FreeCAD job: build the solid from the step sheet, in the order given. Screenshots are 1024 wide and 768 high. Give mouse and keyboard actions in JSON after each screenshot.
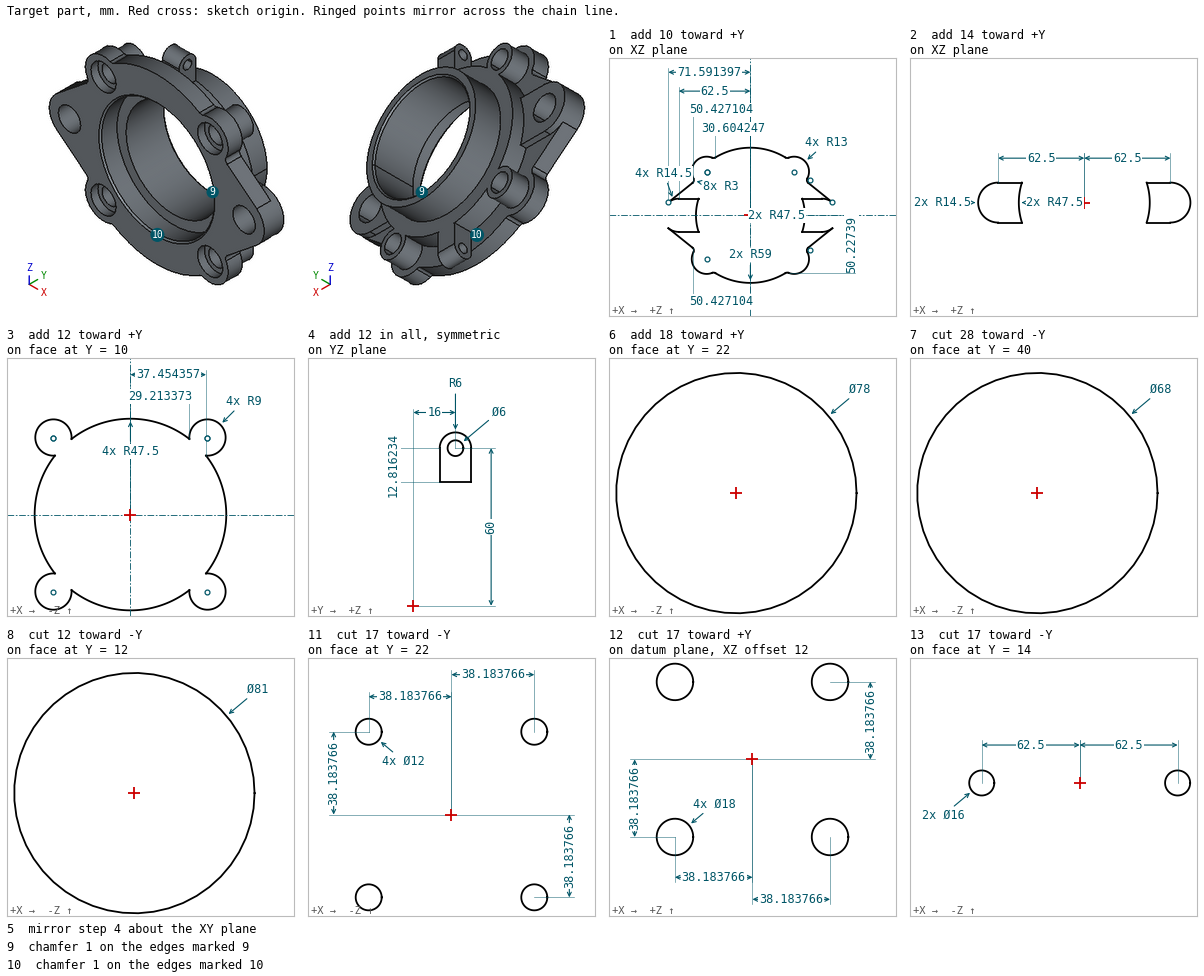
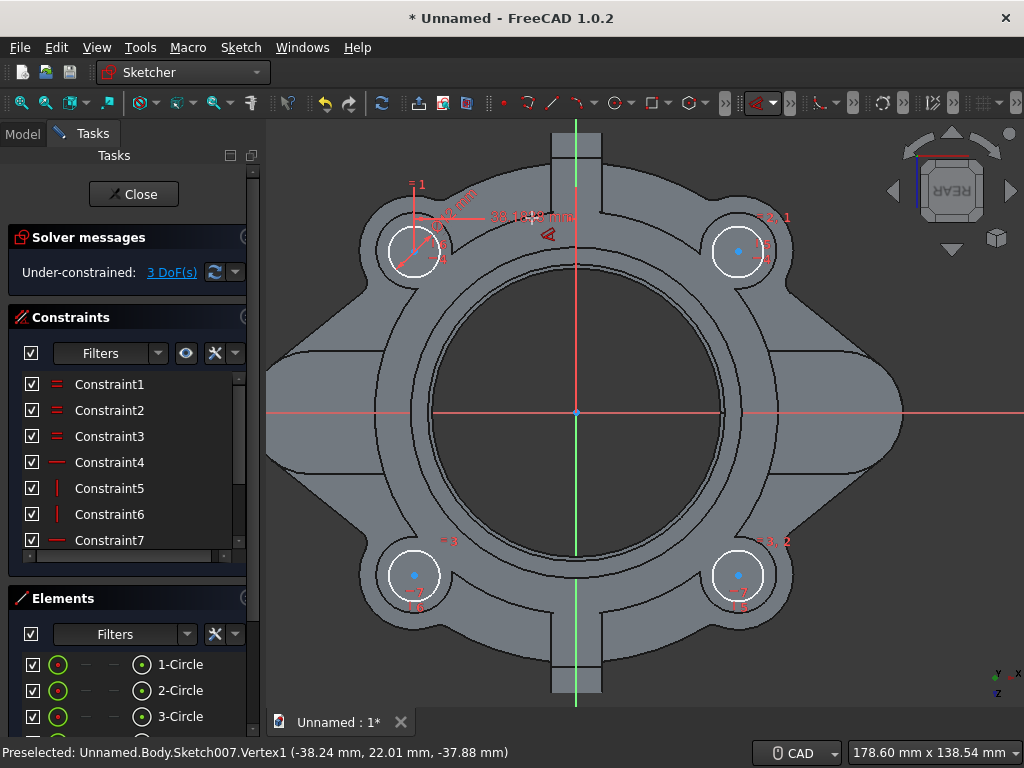
{"action": "left_click", "coordinate": [414, 252]}
{"action": "left_click", "coordinate": [380, 332]}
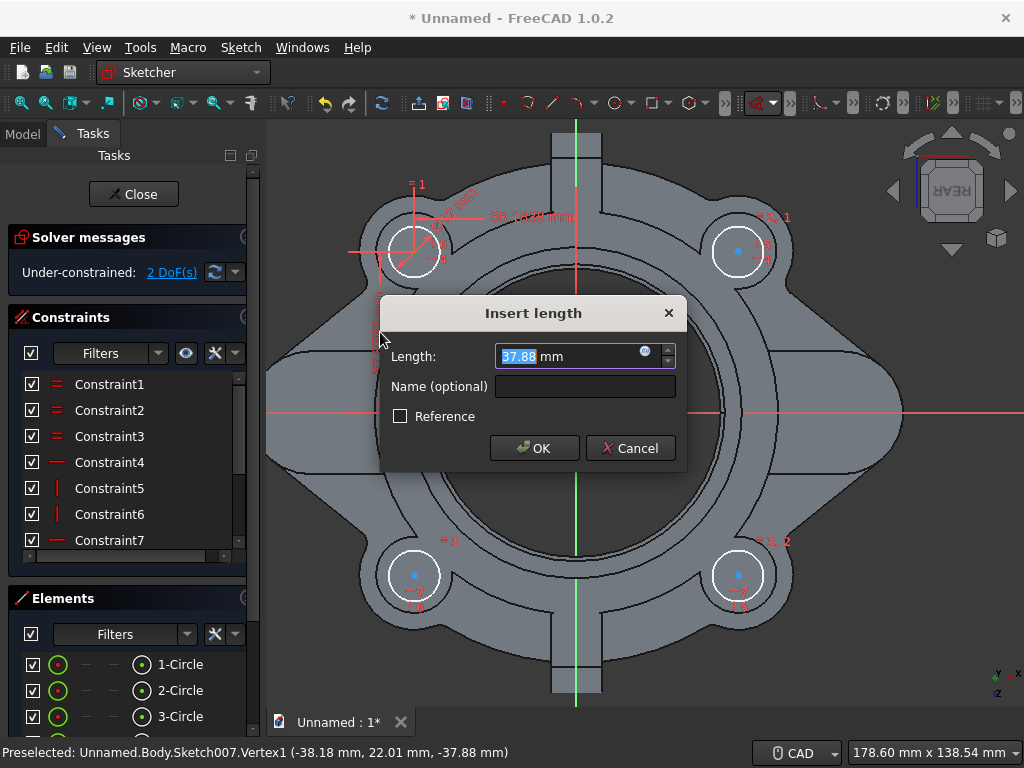
{"action": "type", "text": "38.183766"}
{"action": "key", "text": "Return"}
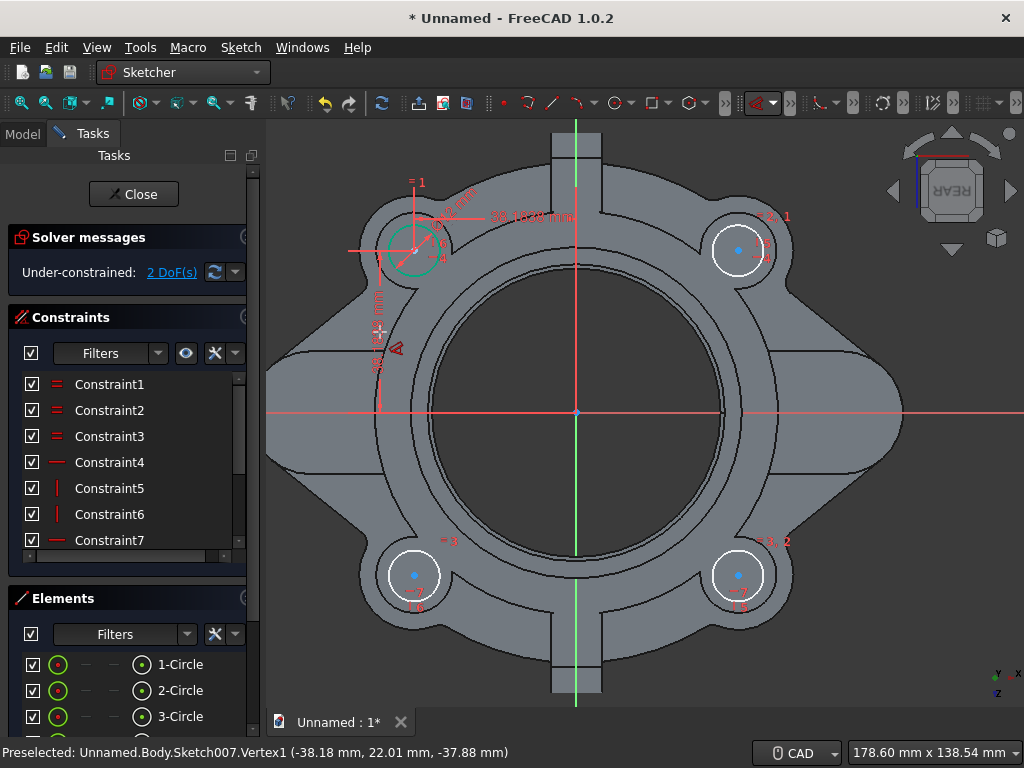
{"action": "left_click", "coordinate": [738, 251]}
{"action": "left_click", "coordinate": [657, 217]}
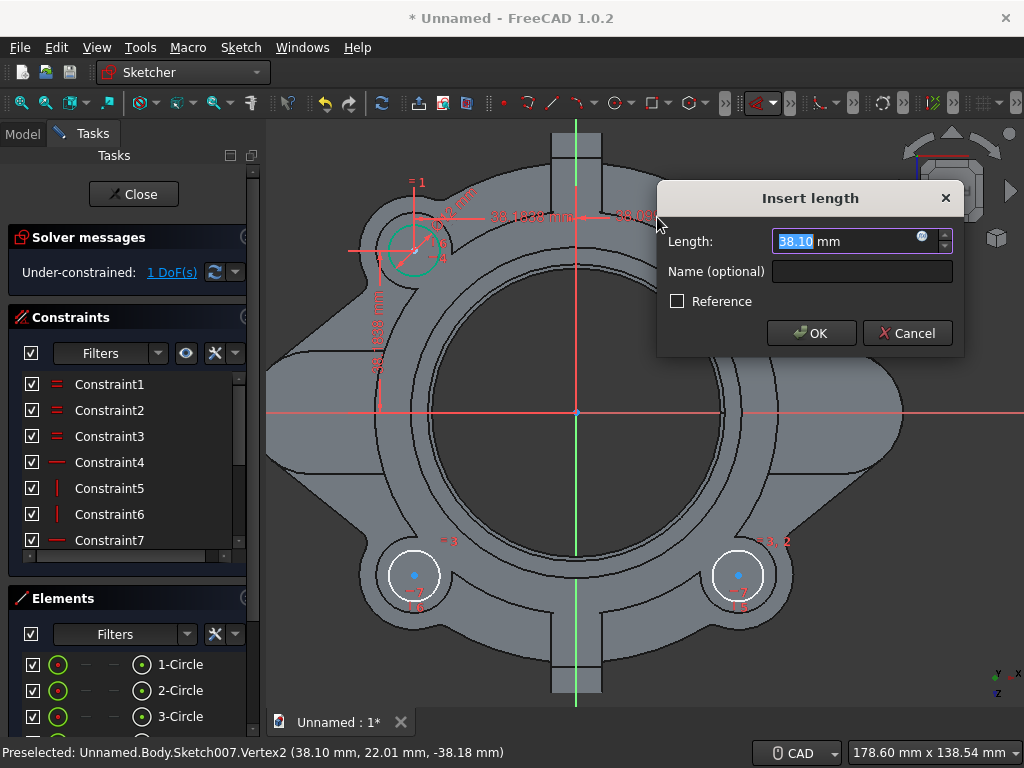
{"action": "type", "text": "38.183766"}
{"action": "key", "text": "Return"}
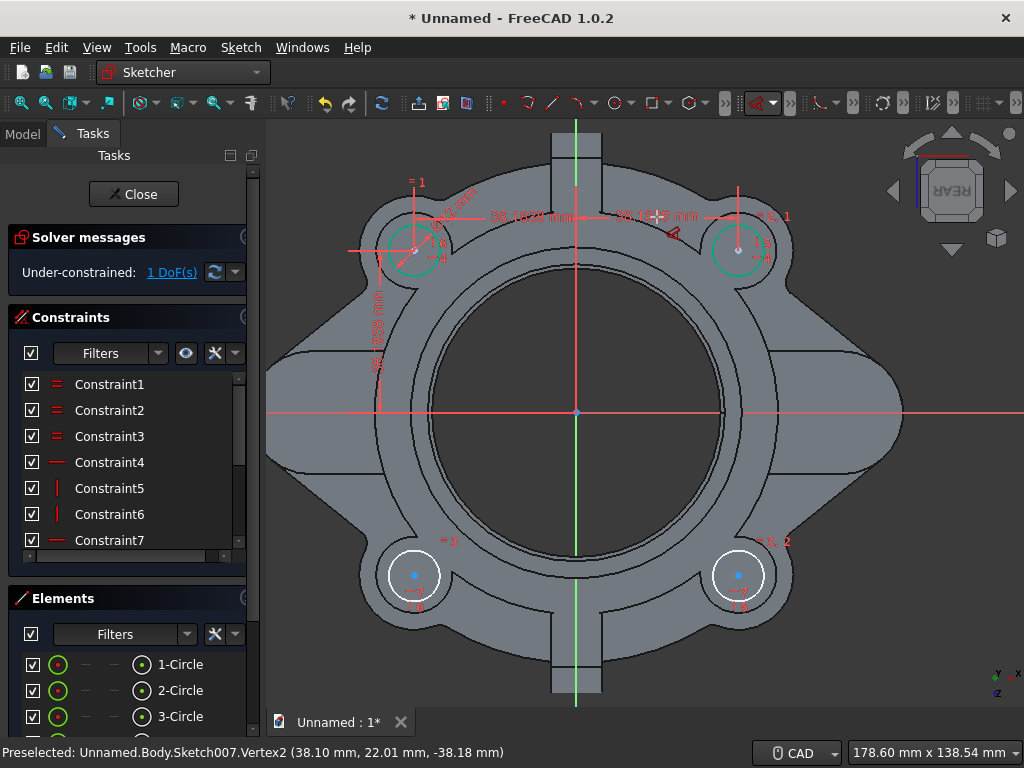
{"action": "left_click", "coordinate": [738, 576]}
{"action": "left_click", "coordinate": [772, 494]}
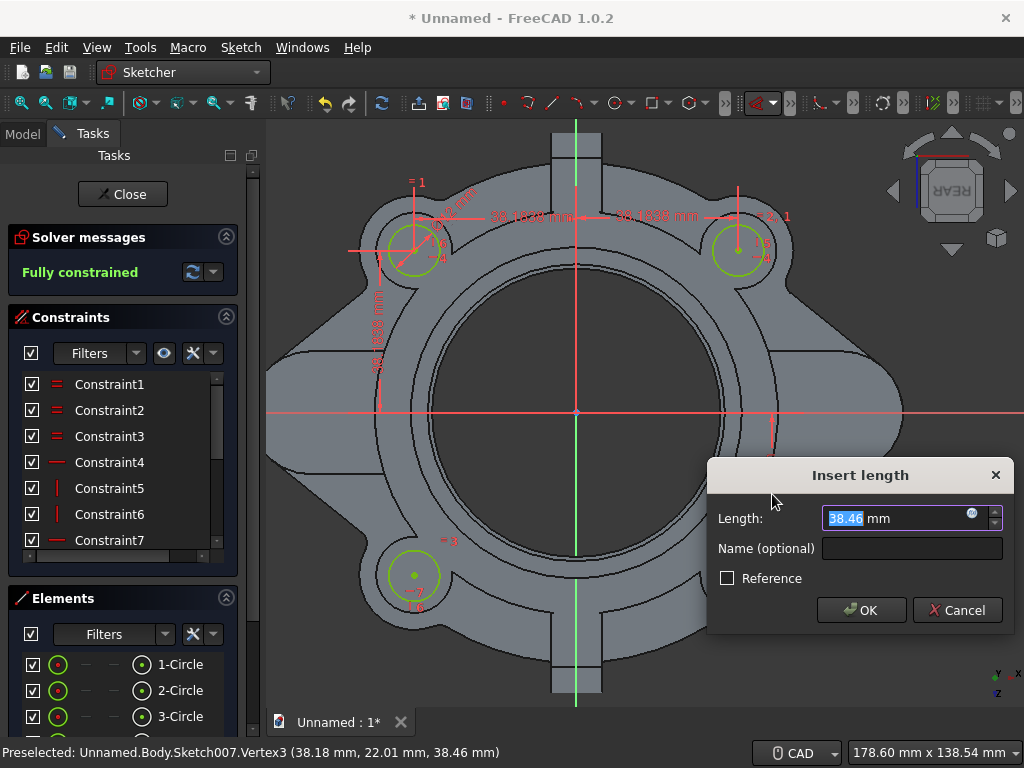
{"action": "type", "text": "38.183766"}
{"action": "key", "text": "Return"}
{"action": "key", "text": "Escape"}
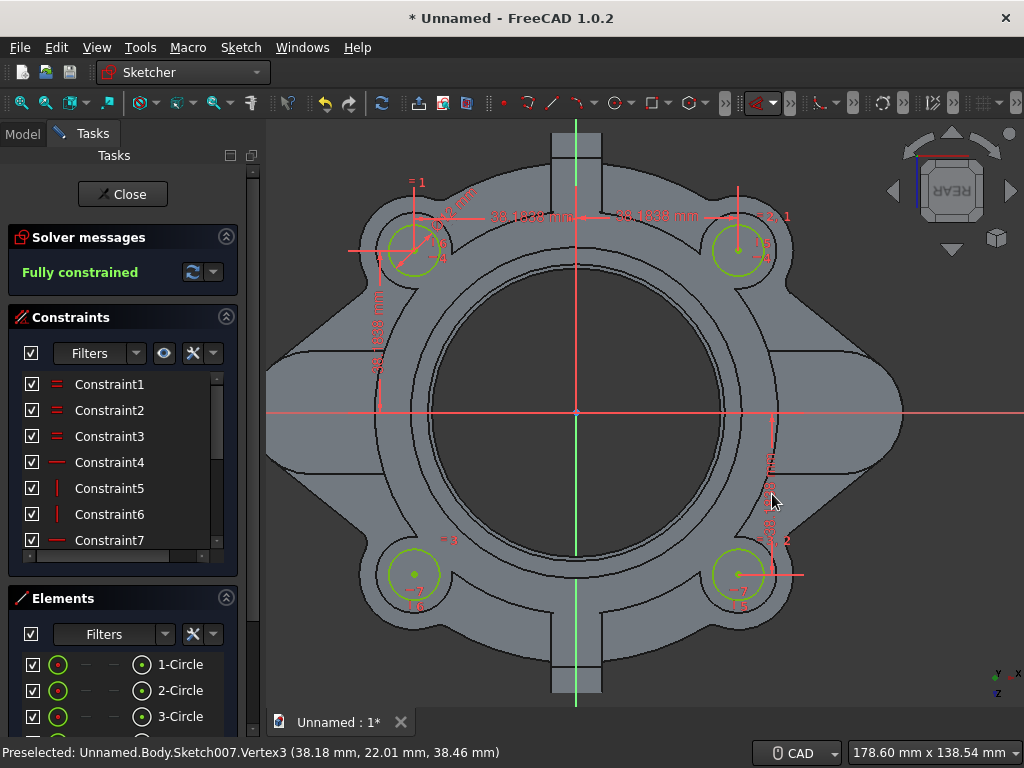
{"action": "left_click", "coordinate": [123, 194]}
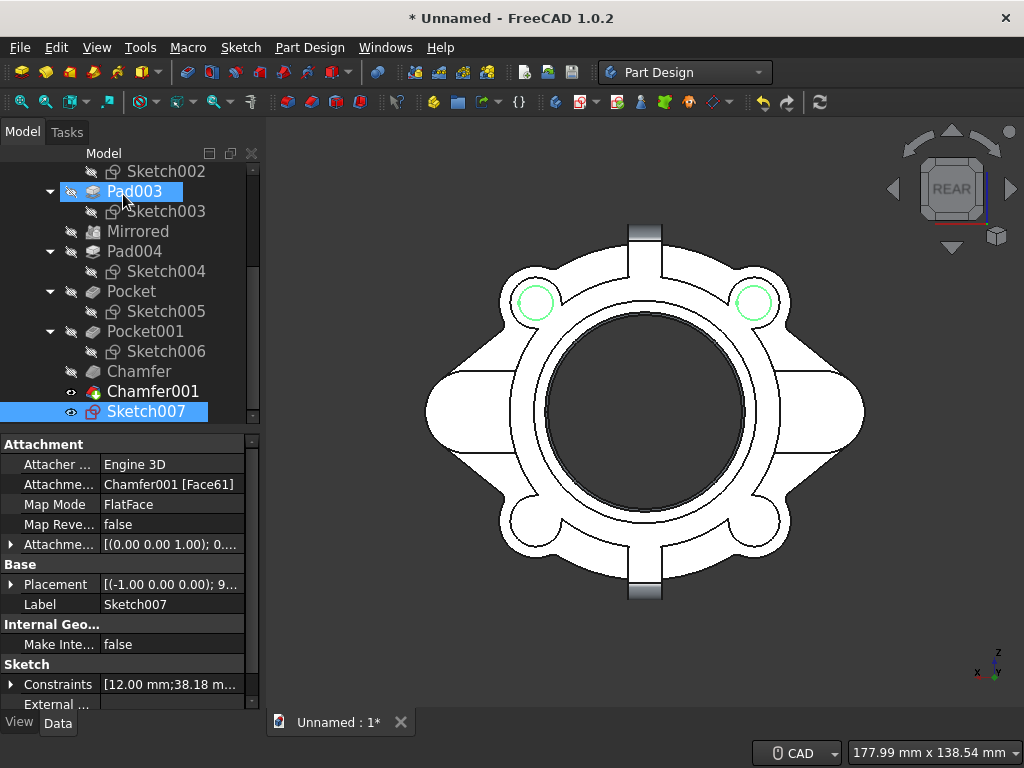
{"action": "left_click", "coordinate": [188, 72]}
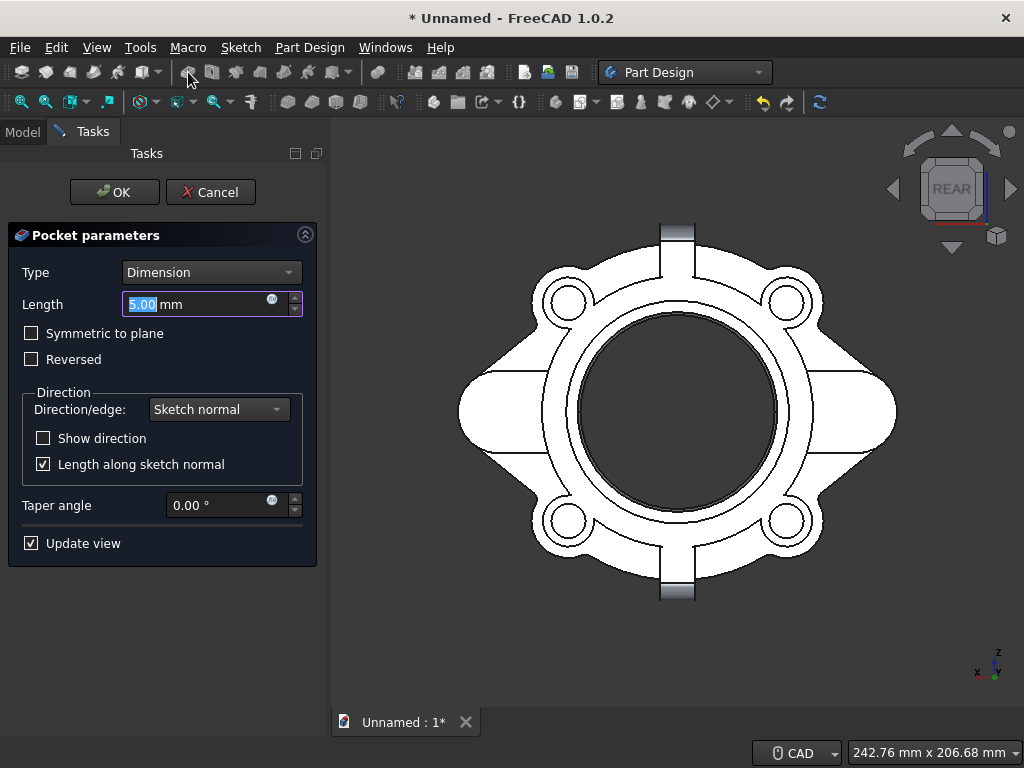
{"action": "type", "text": "17"}
{"action": "key", "text": "Tab"}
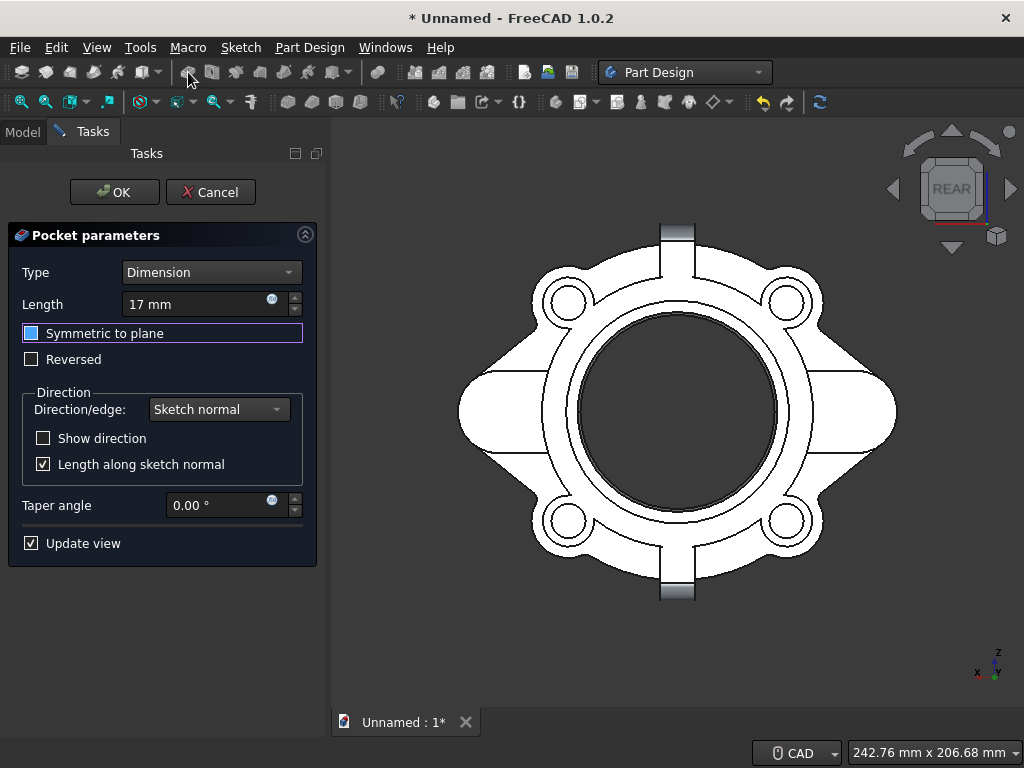
{"action": "left_click", "coordinate": [115, 192]}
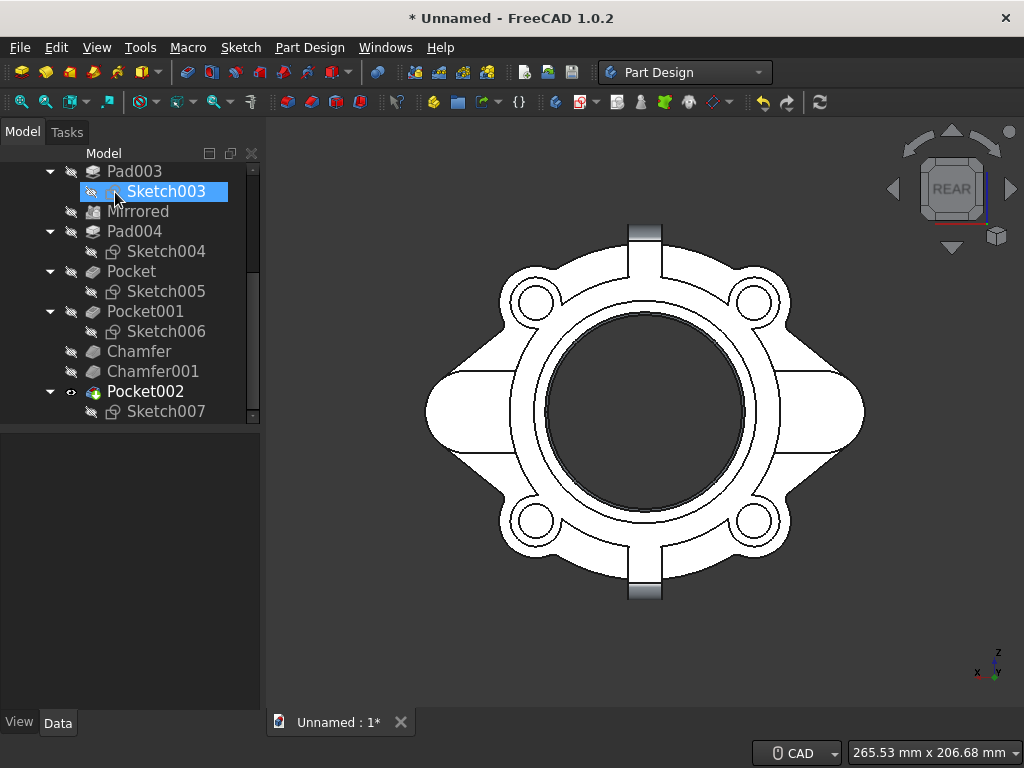
{"action": "scroll", "coordinate": [140, 287], "scroll_direction": "down", "scroll_amount": 3}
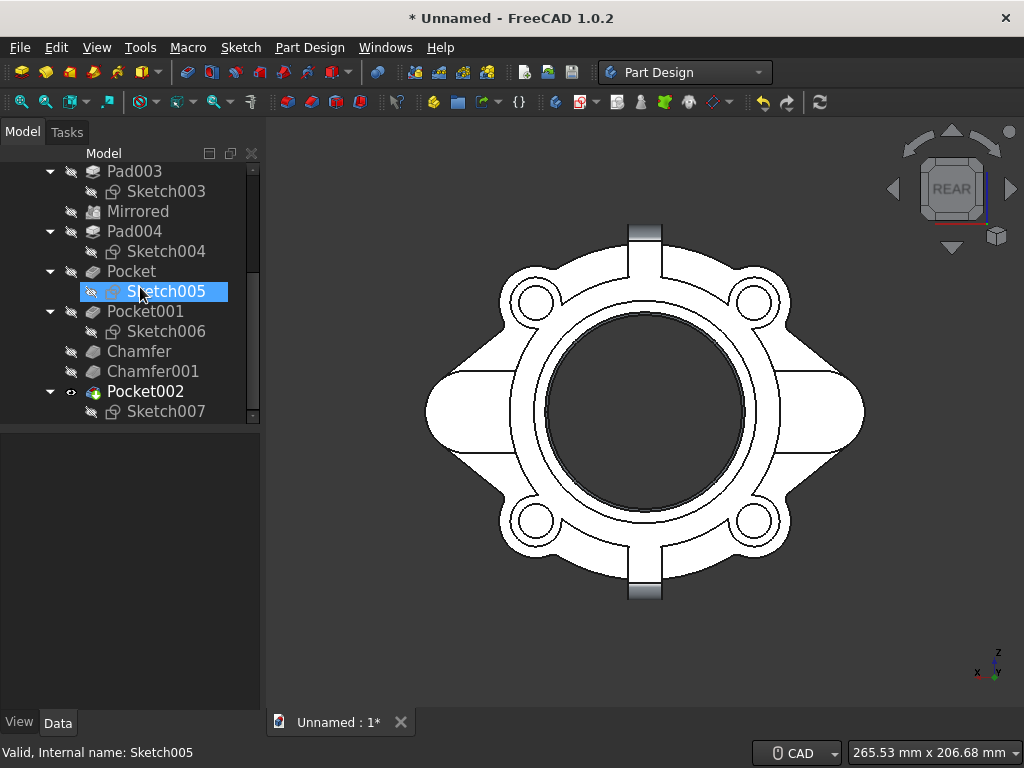
{"action": "scroll", "coordinate": [140, 287], "scroll_direction": "up", "scroll_amount": 15}